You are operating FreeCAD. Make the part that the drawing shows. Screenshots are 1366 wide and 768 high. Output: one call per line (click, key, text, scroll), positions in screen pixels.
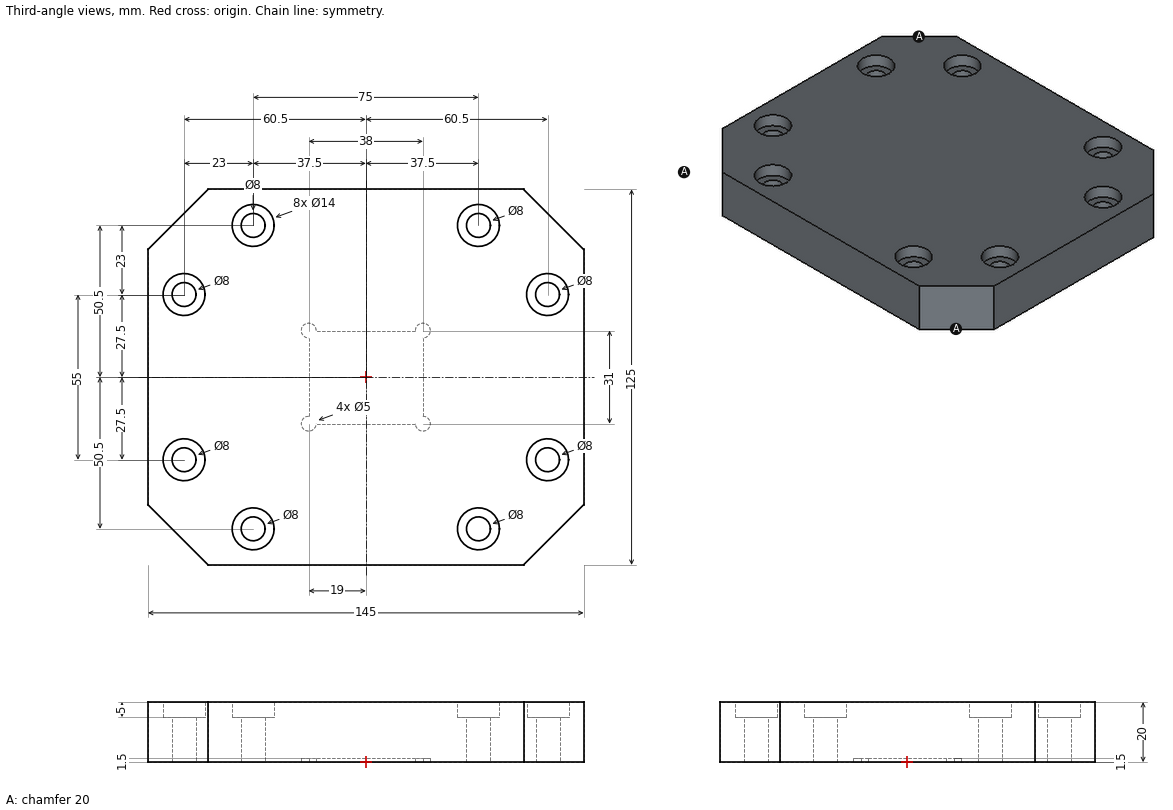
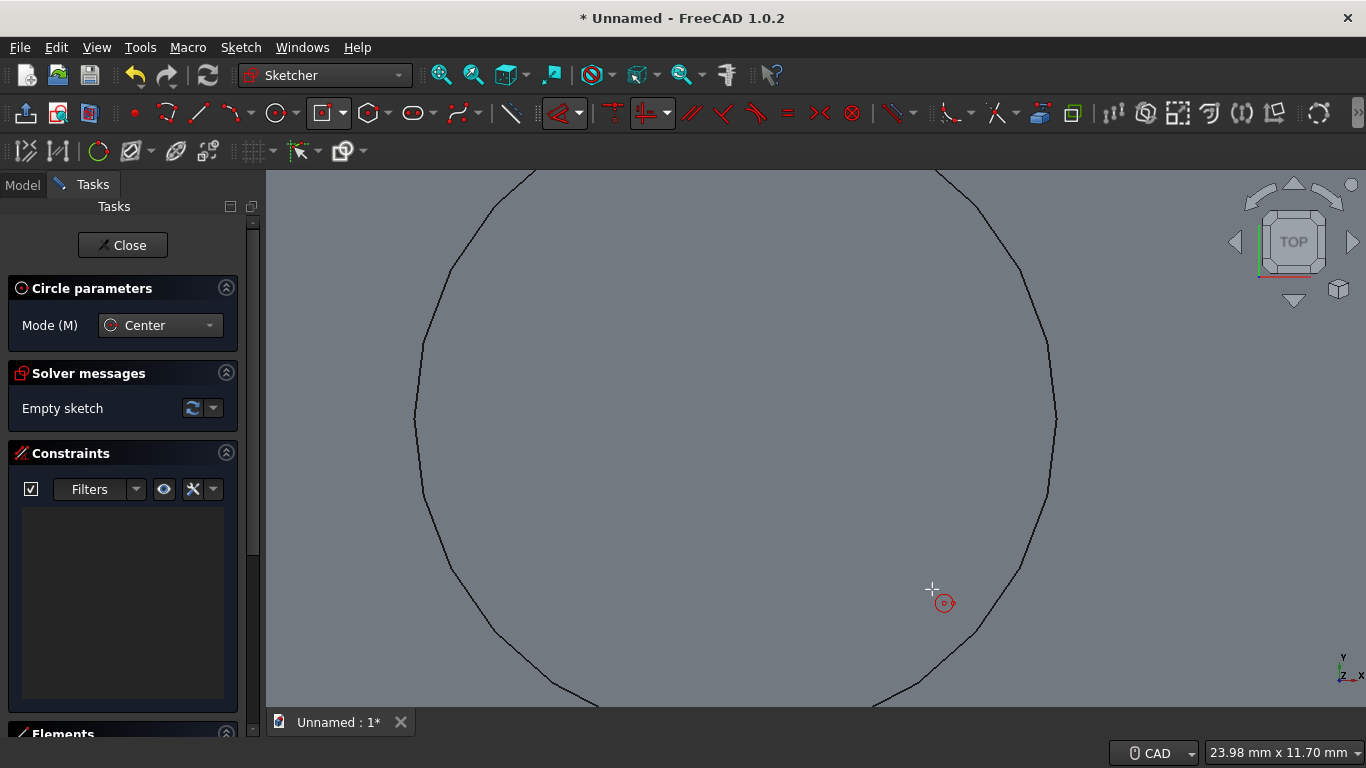
click(735, 419)
click(865, 289)
key(Escape)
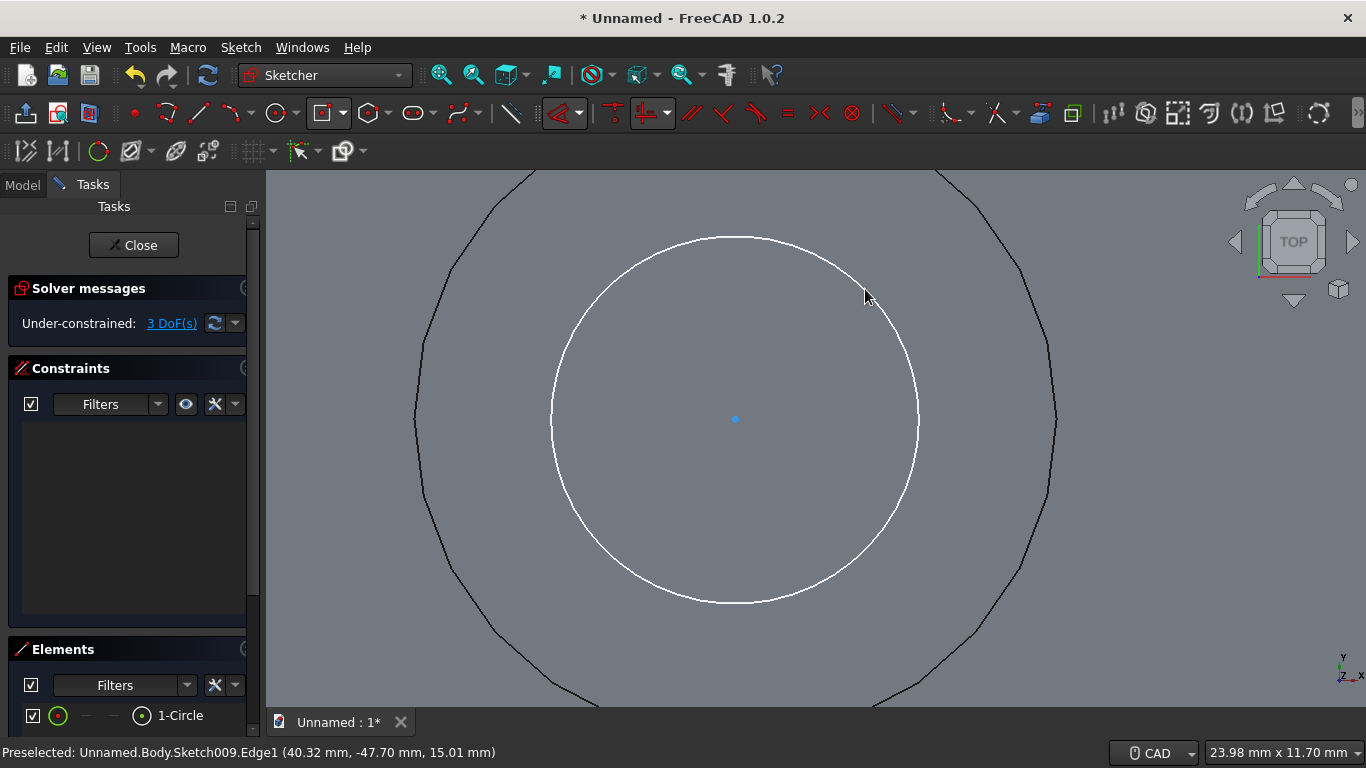
click(865, 290)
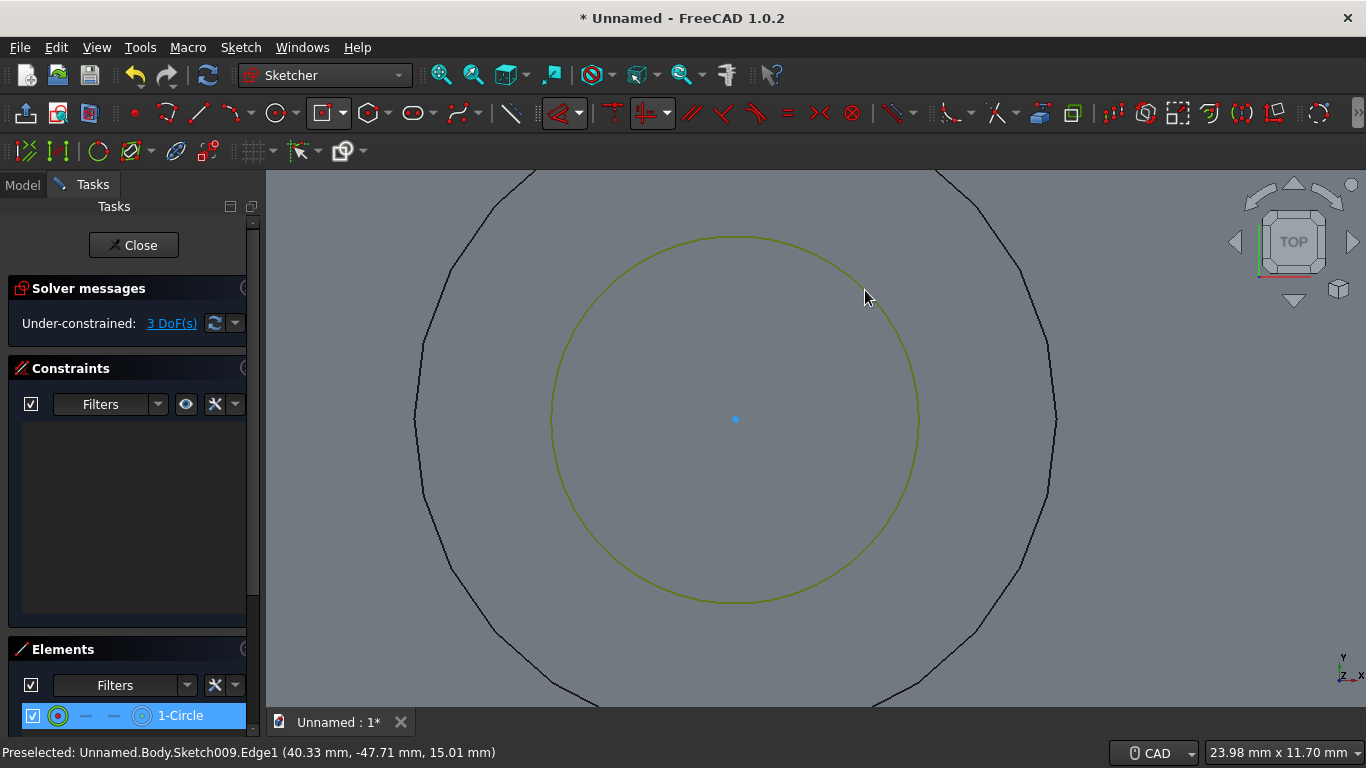
key(k)
key(o)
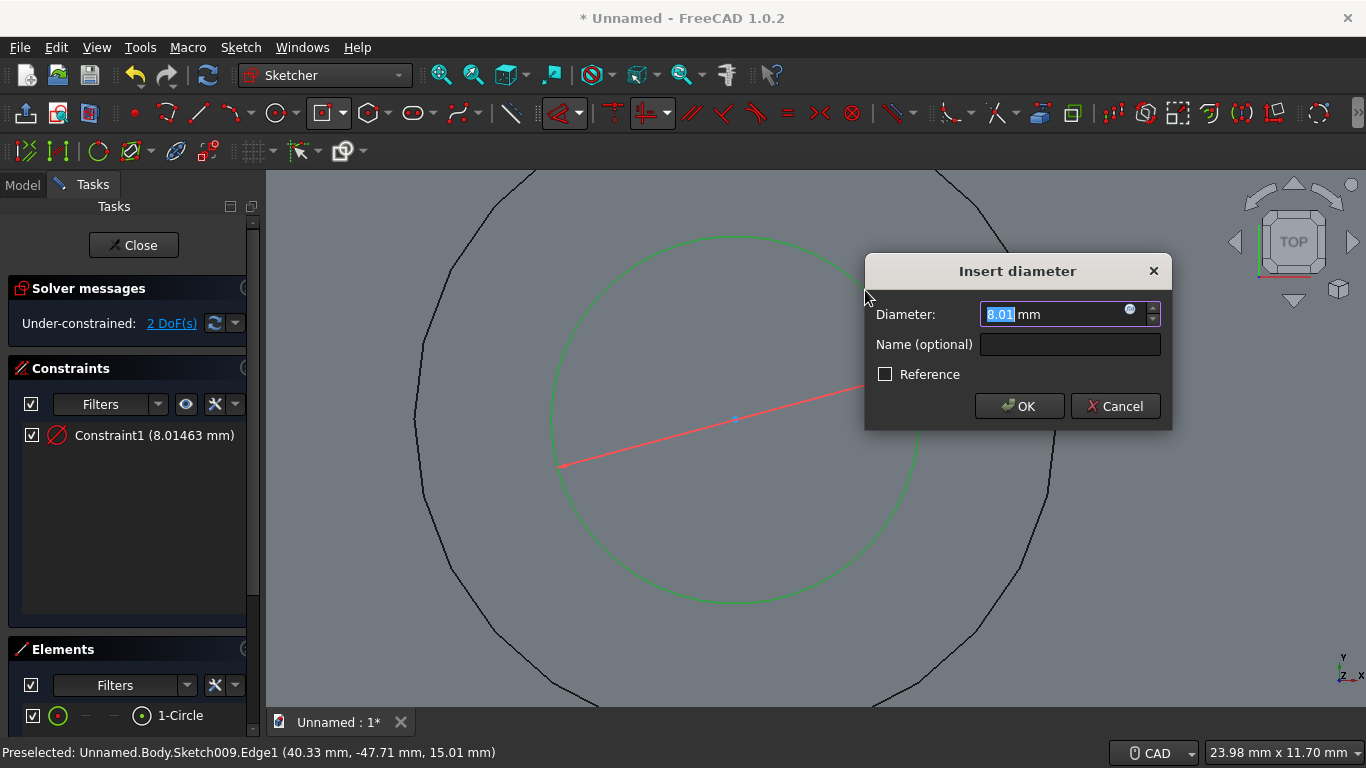
text(8)
key(Return)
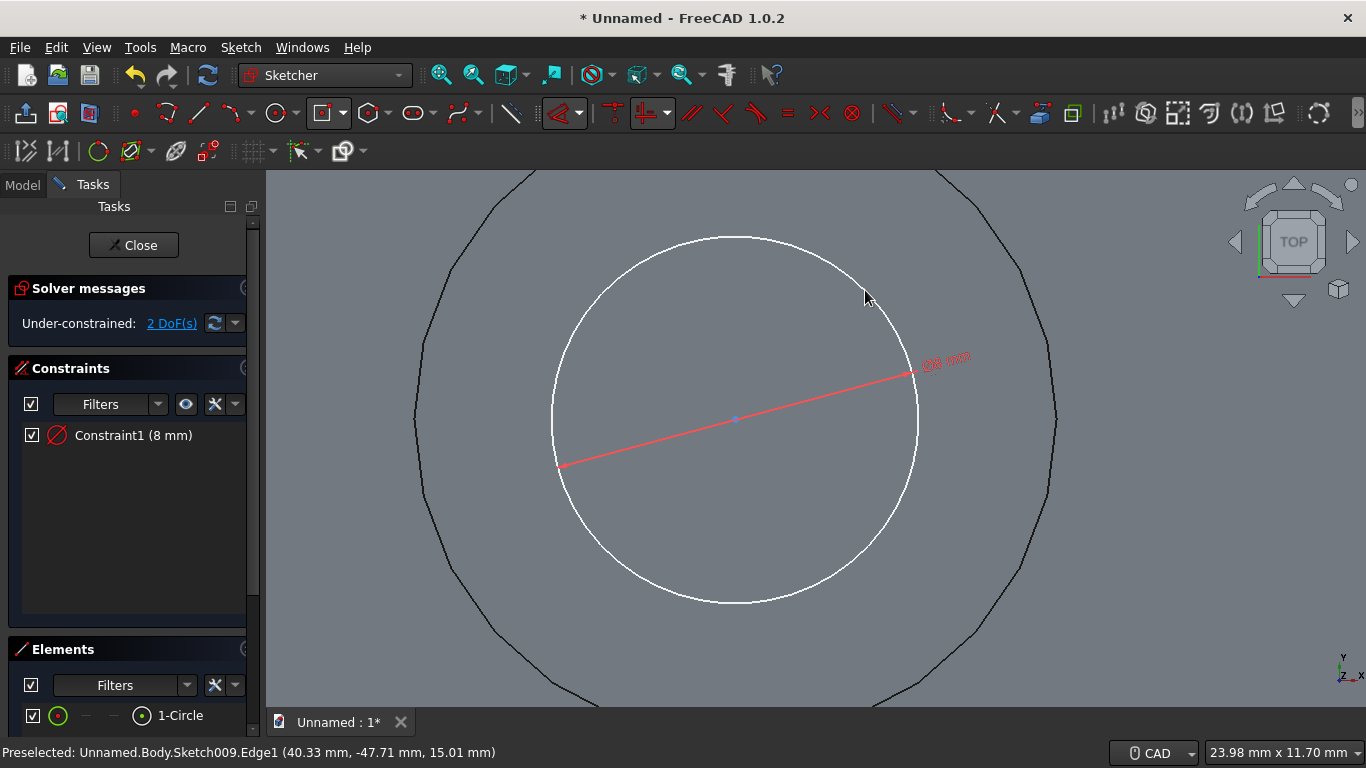
click(735, 420)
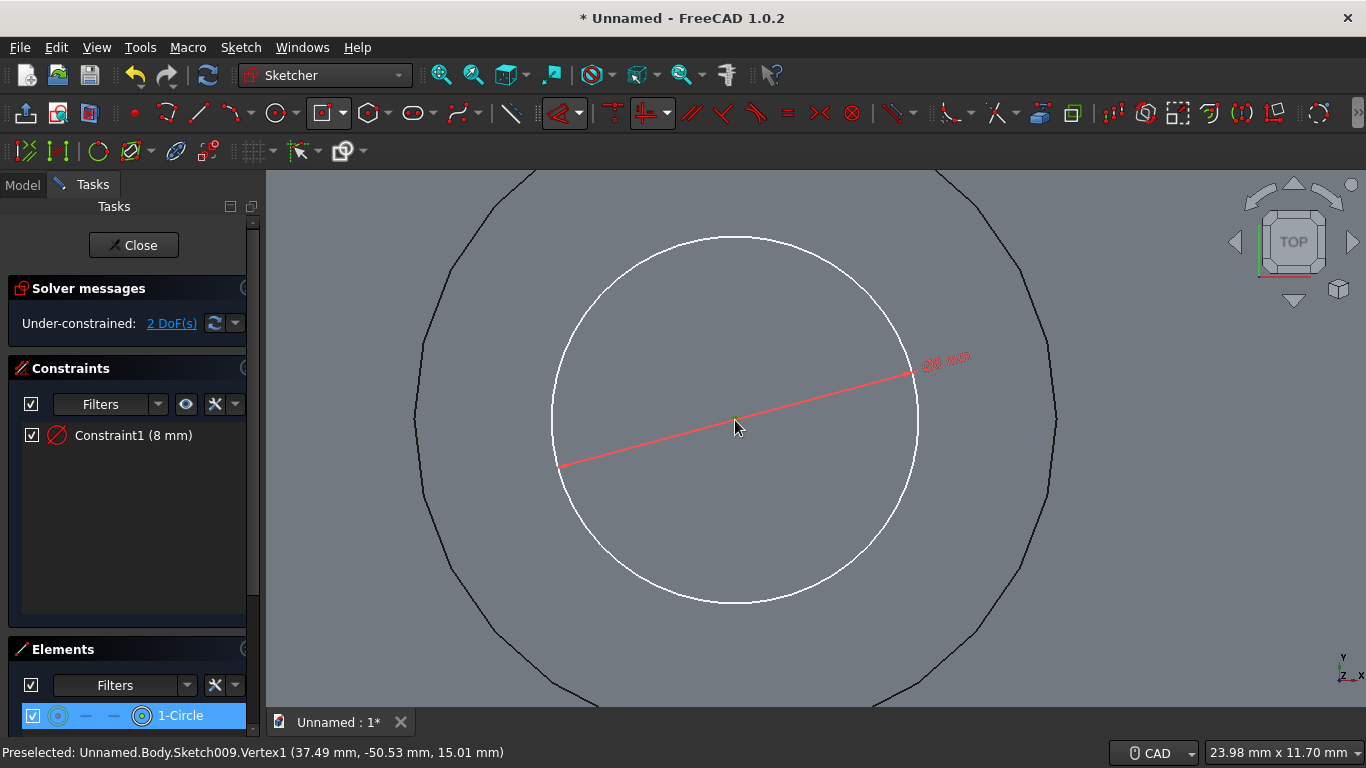
key(l)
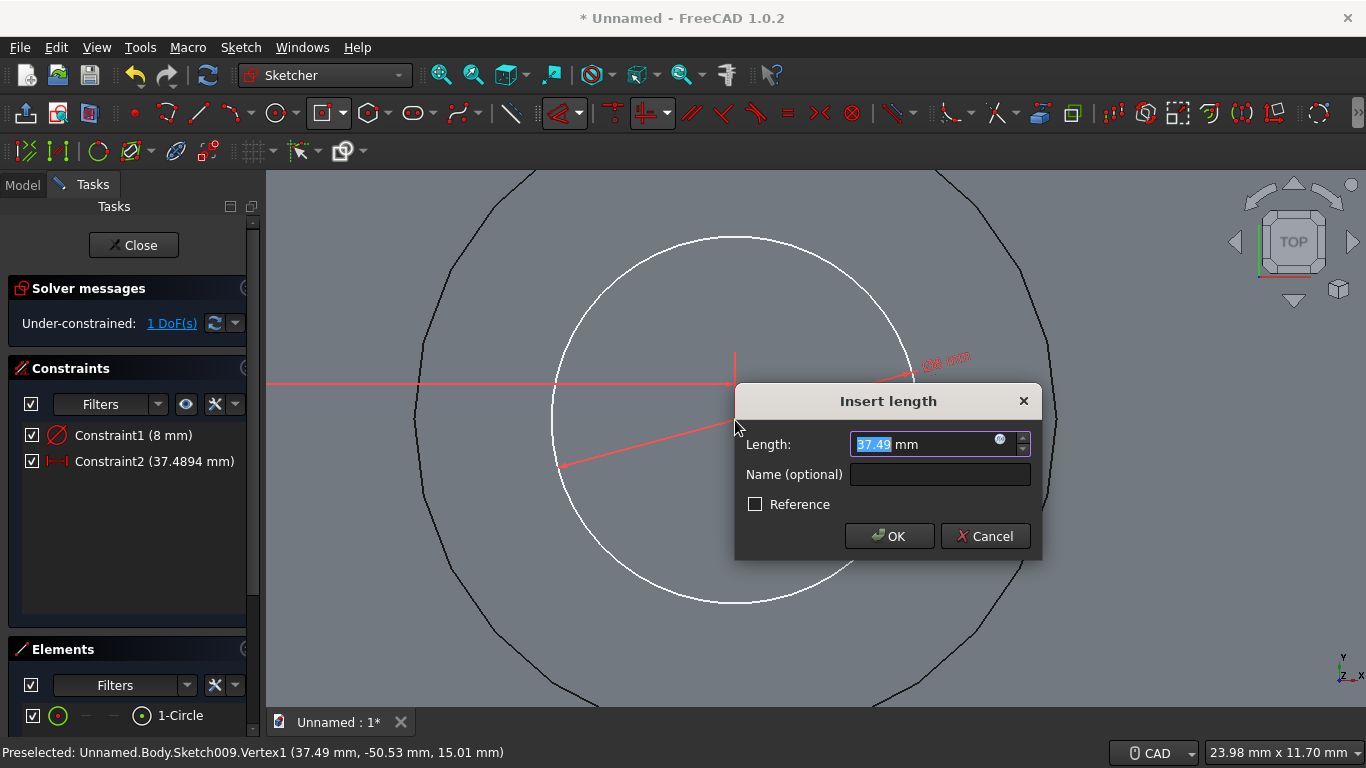
text(37.5)
key(Return)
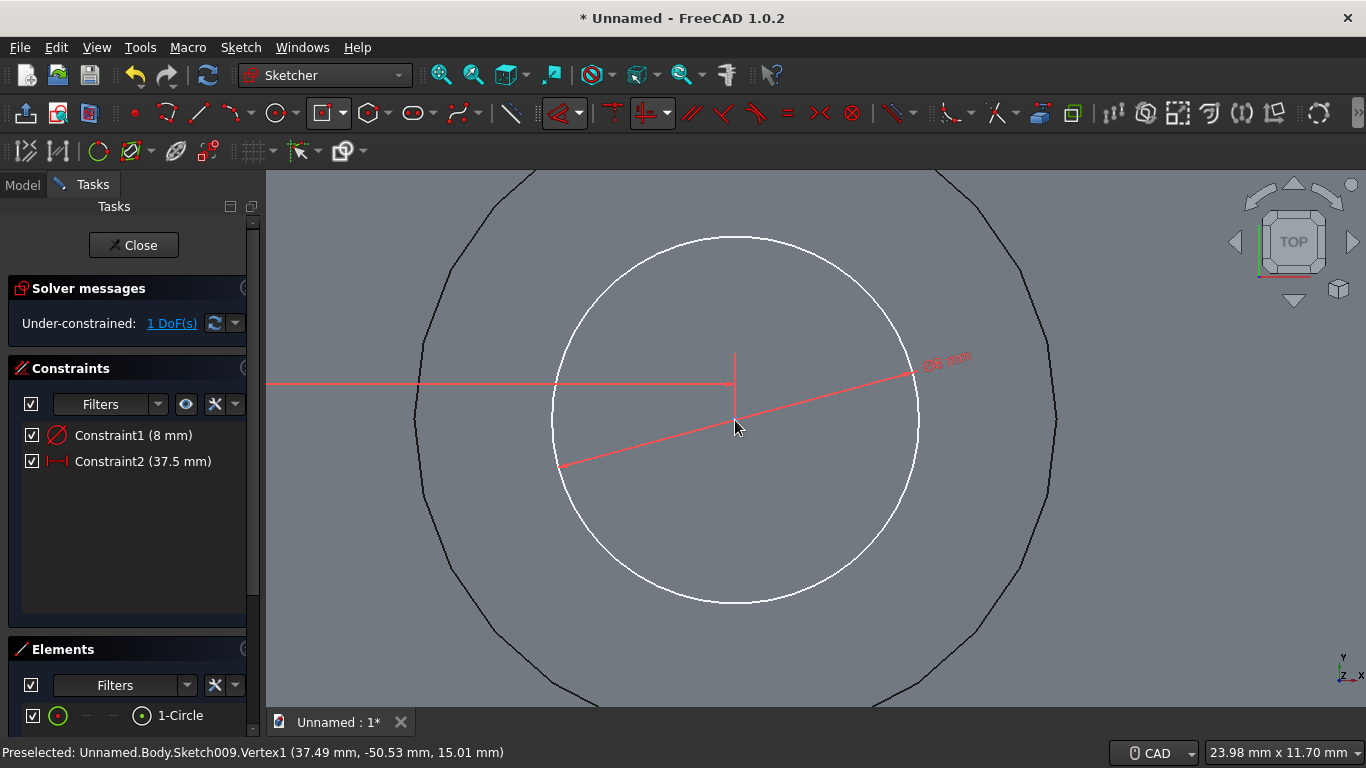
click(735, 420)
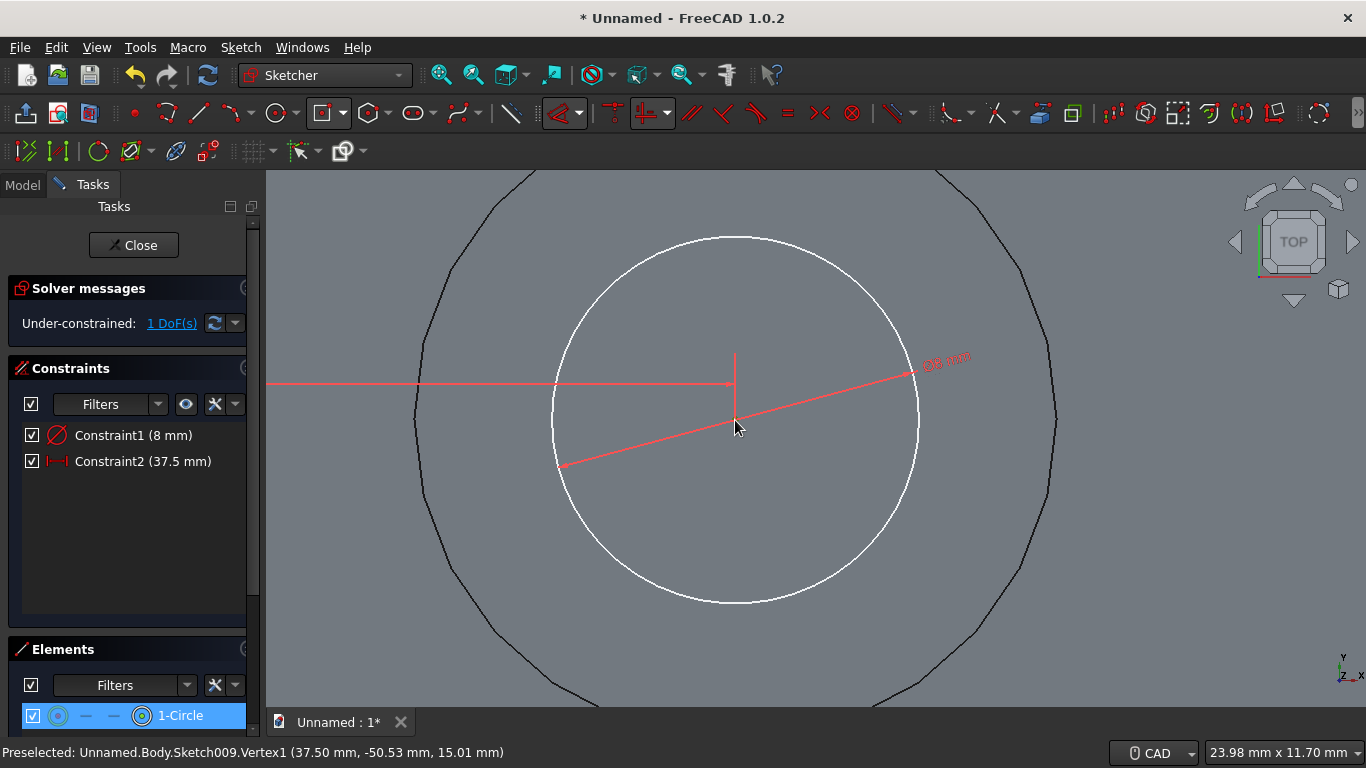
key(i)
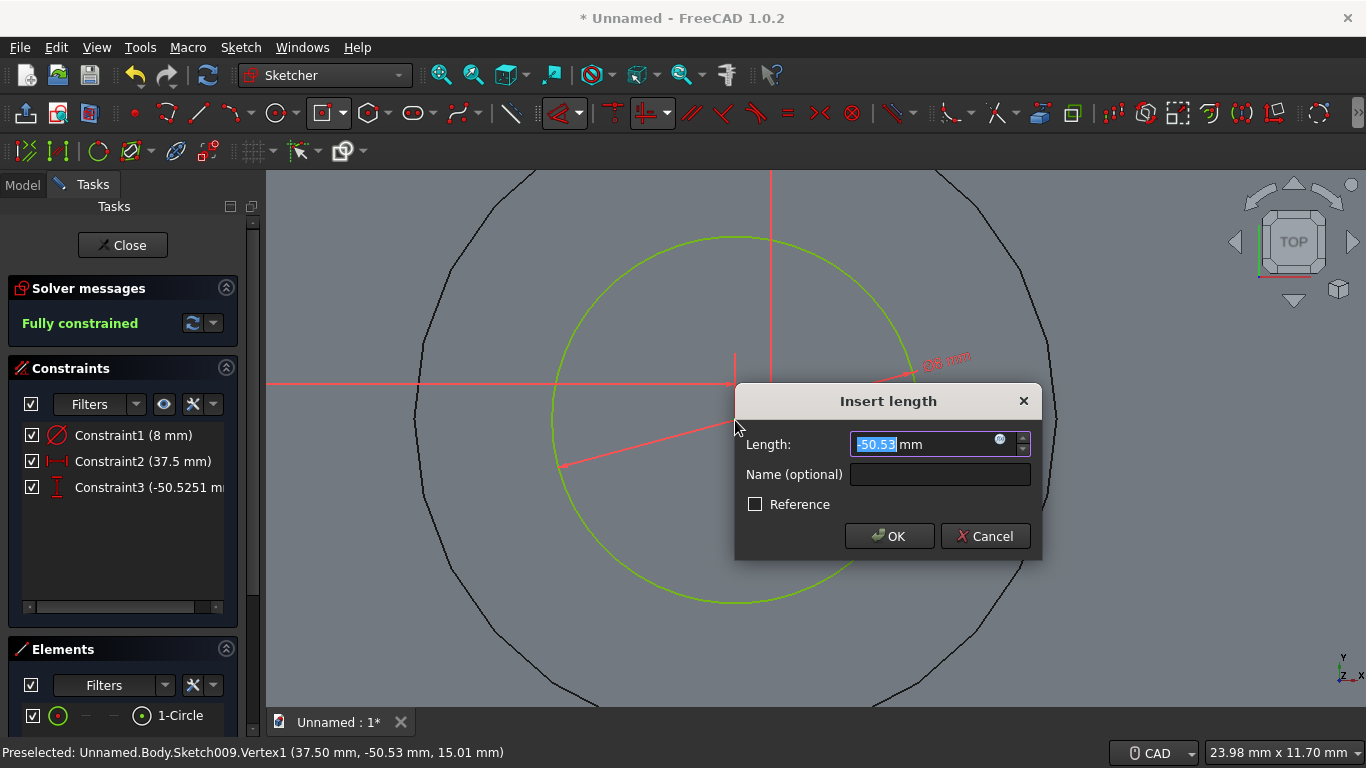
text(-50.5)
key(Return)